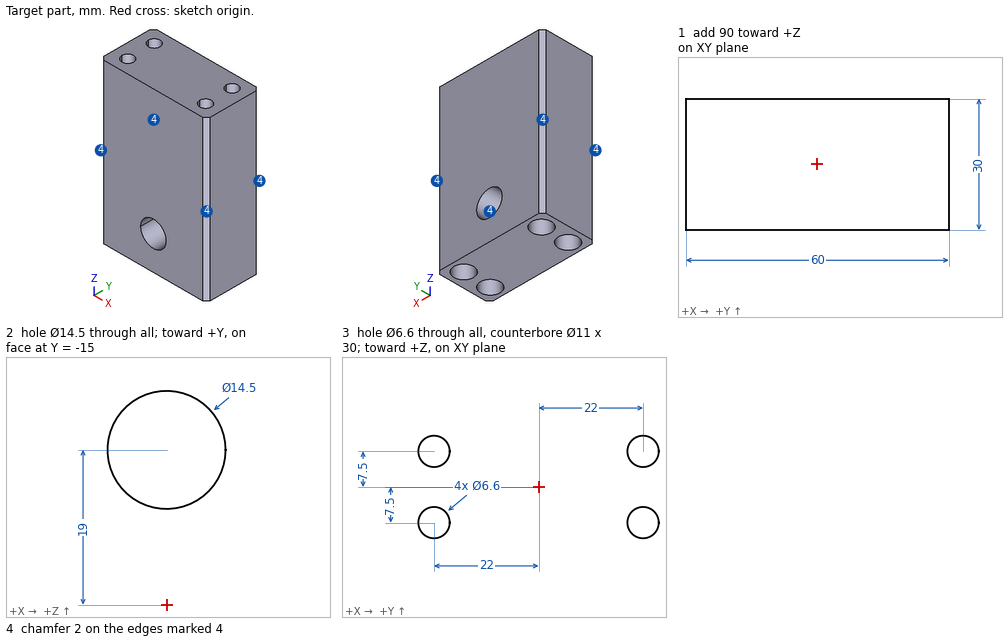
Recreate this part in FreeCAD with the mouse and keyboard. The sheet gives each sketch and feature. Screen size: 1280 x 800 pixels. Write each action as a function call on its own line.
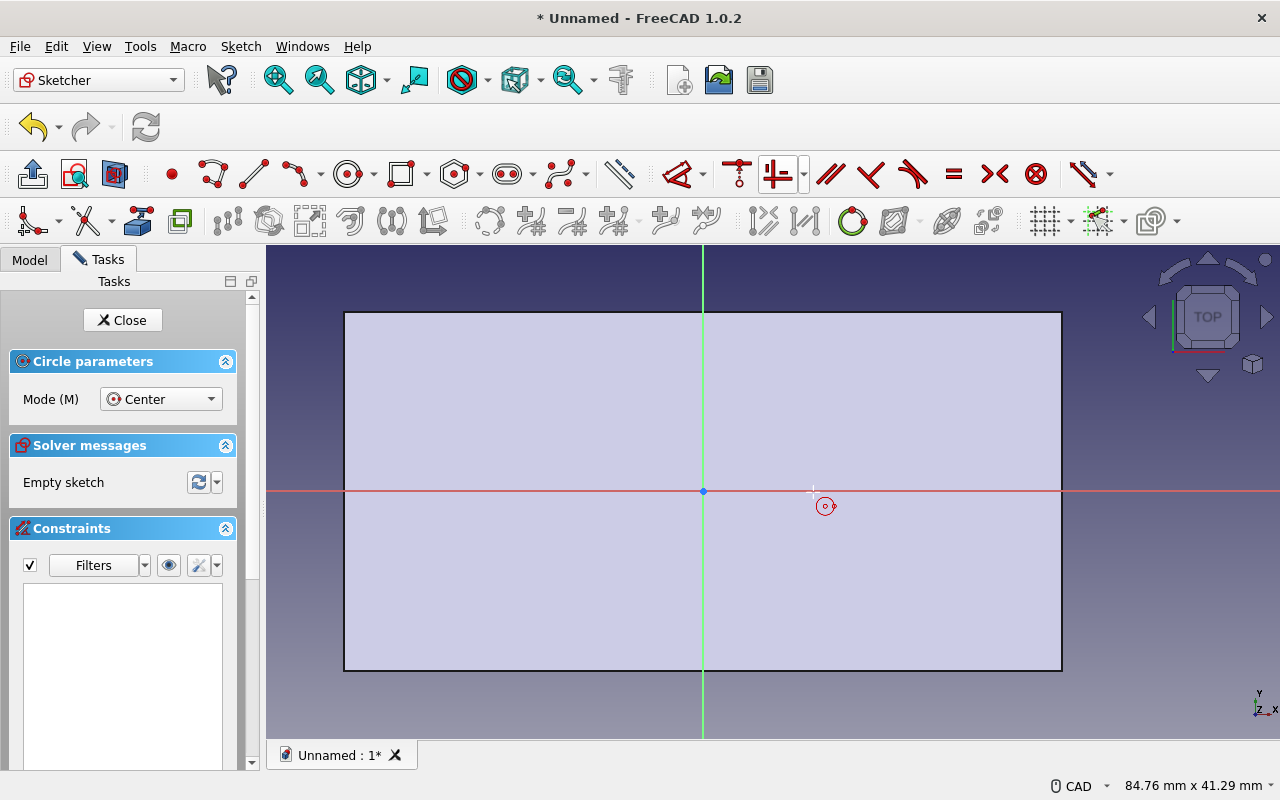
click(440, 581)
click(468, 553)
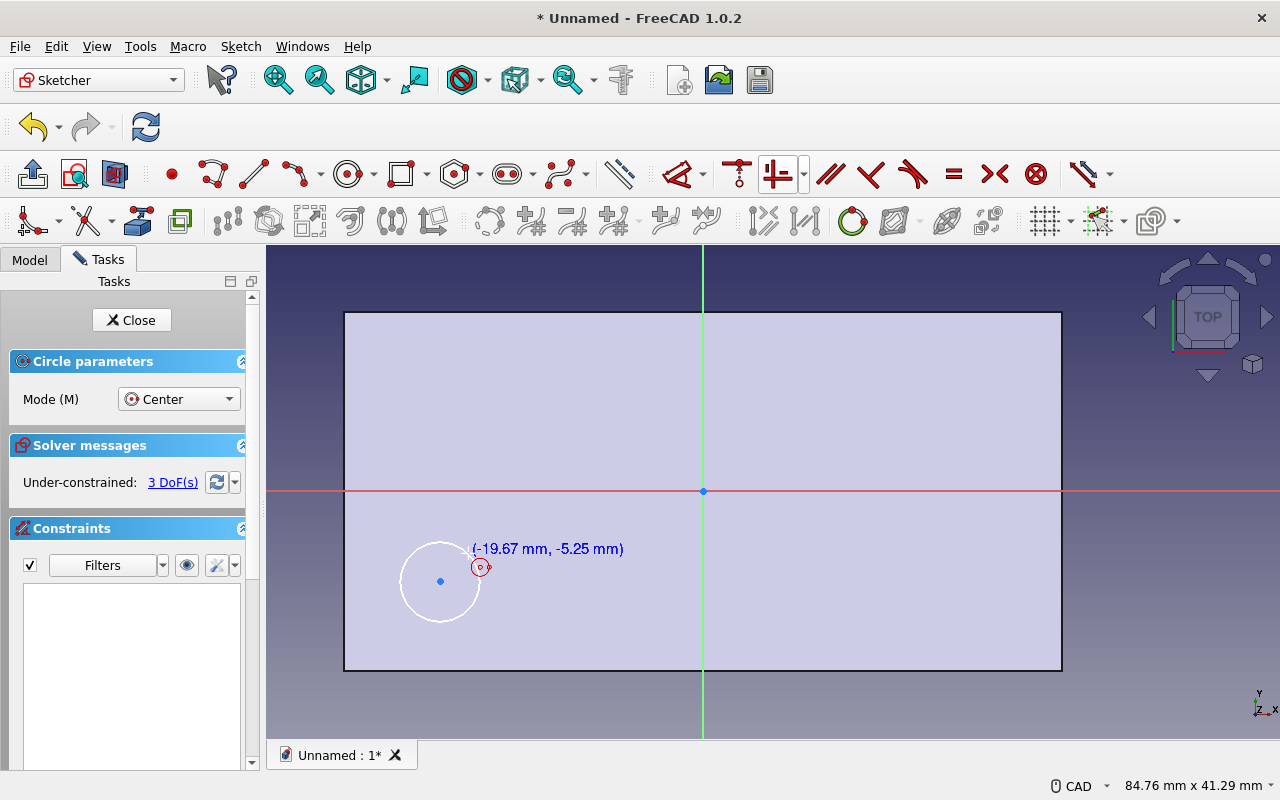
click(440, 401)
click(468, 374)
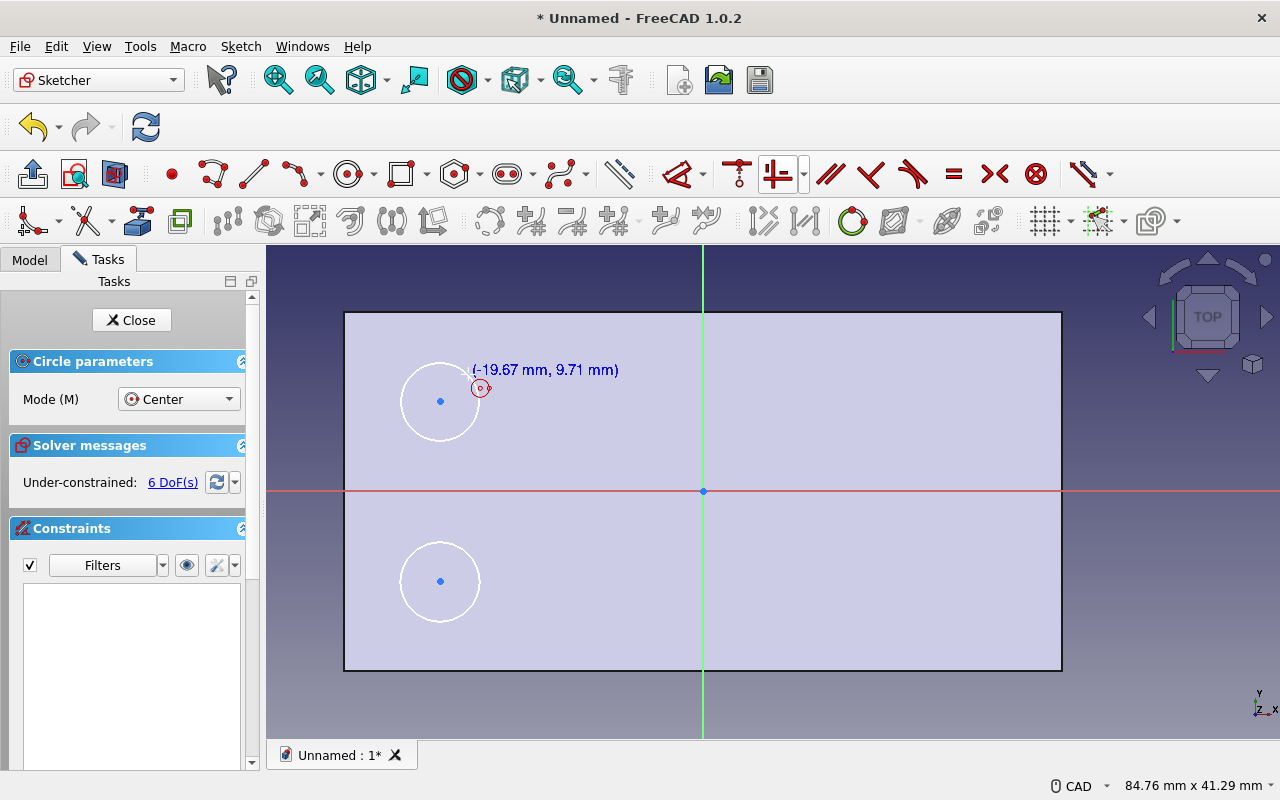
click(967, 401)
click(994, 374)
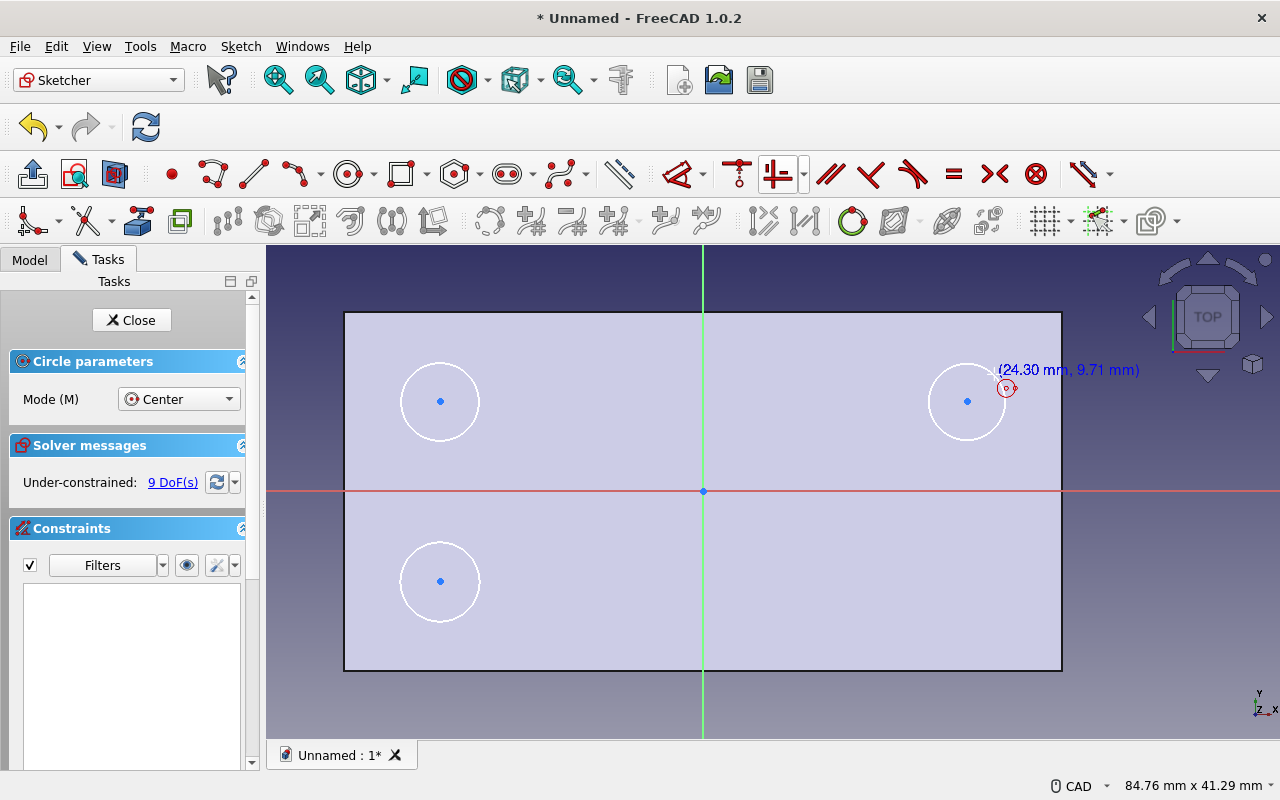
click(967, 581)
click(994, 553)
key(Escape)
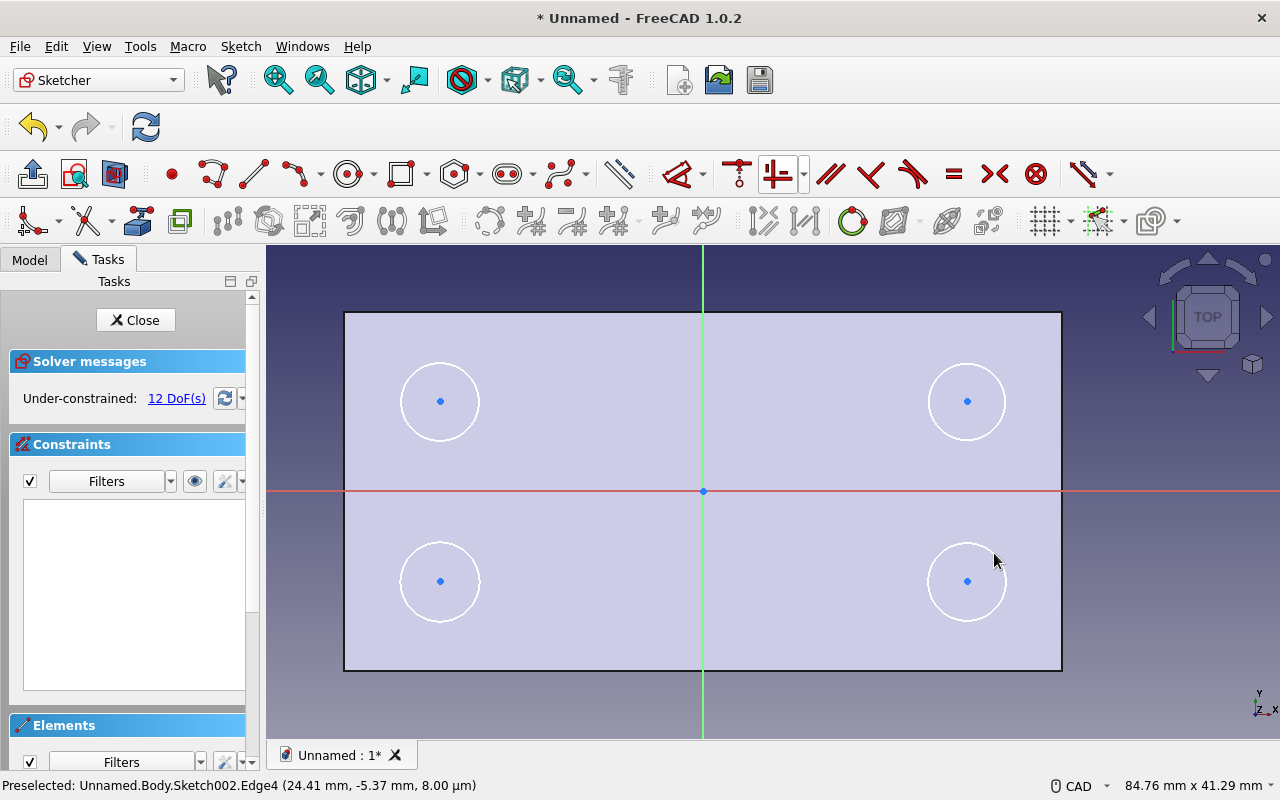
click(468, 554)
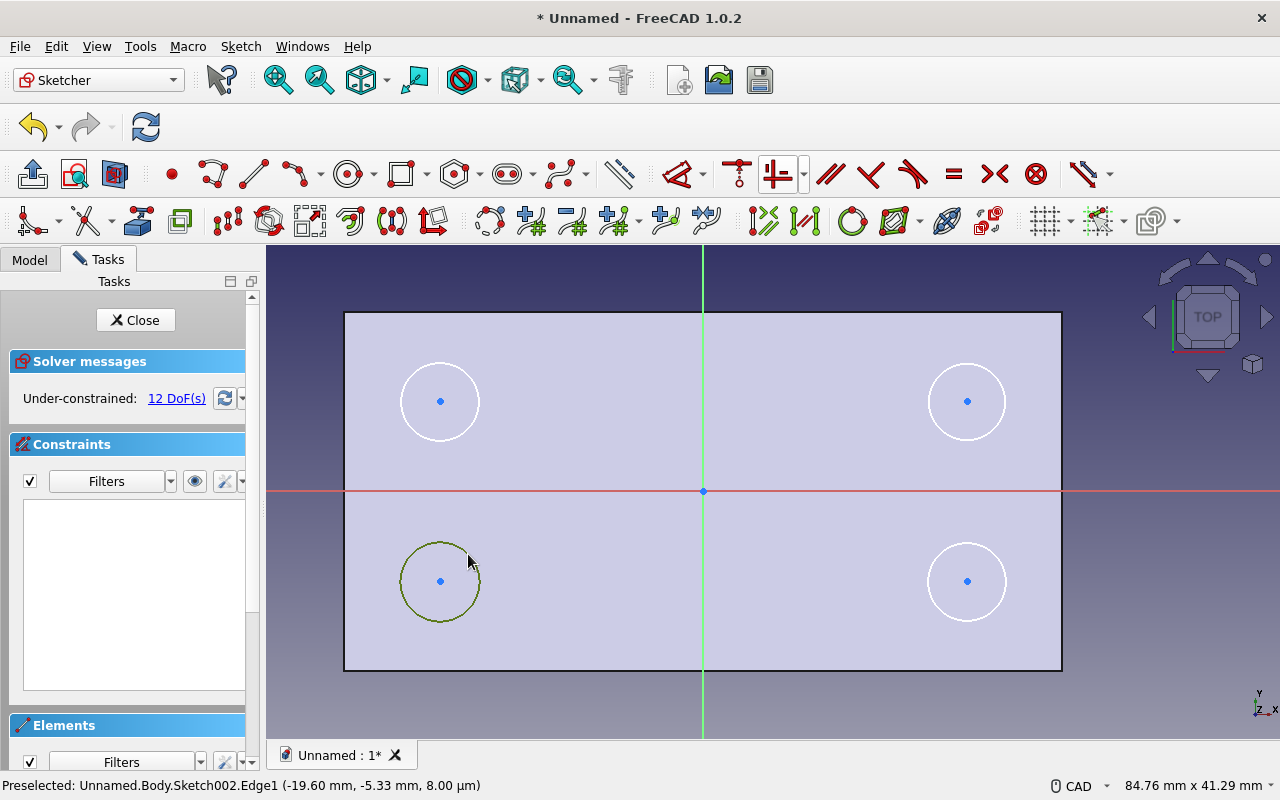
click(467, 374)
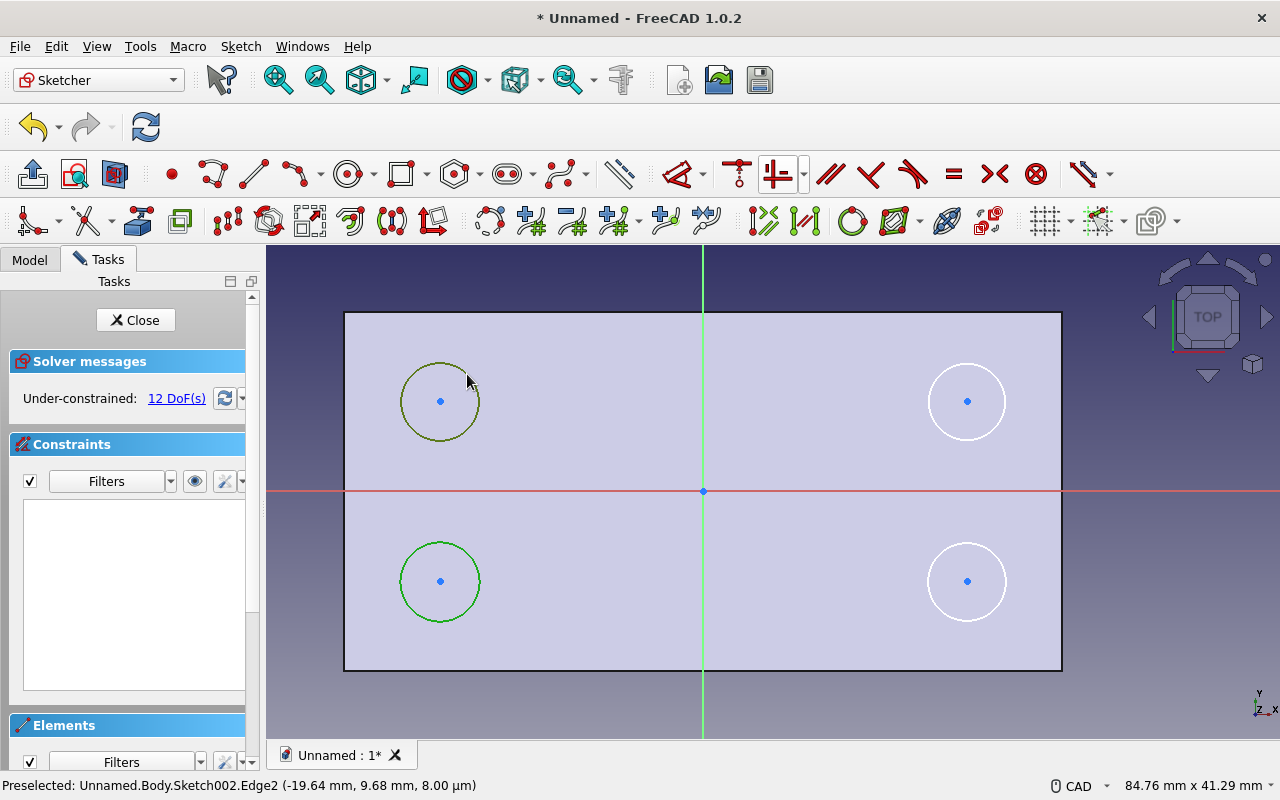
click(994, 375)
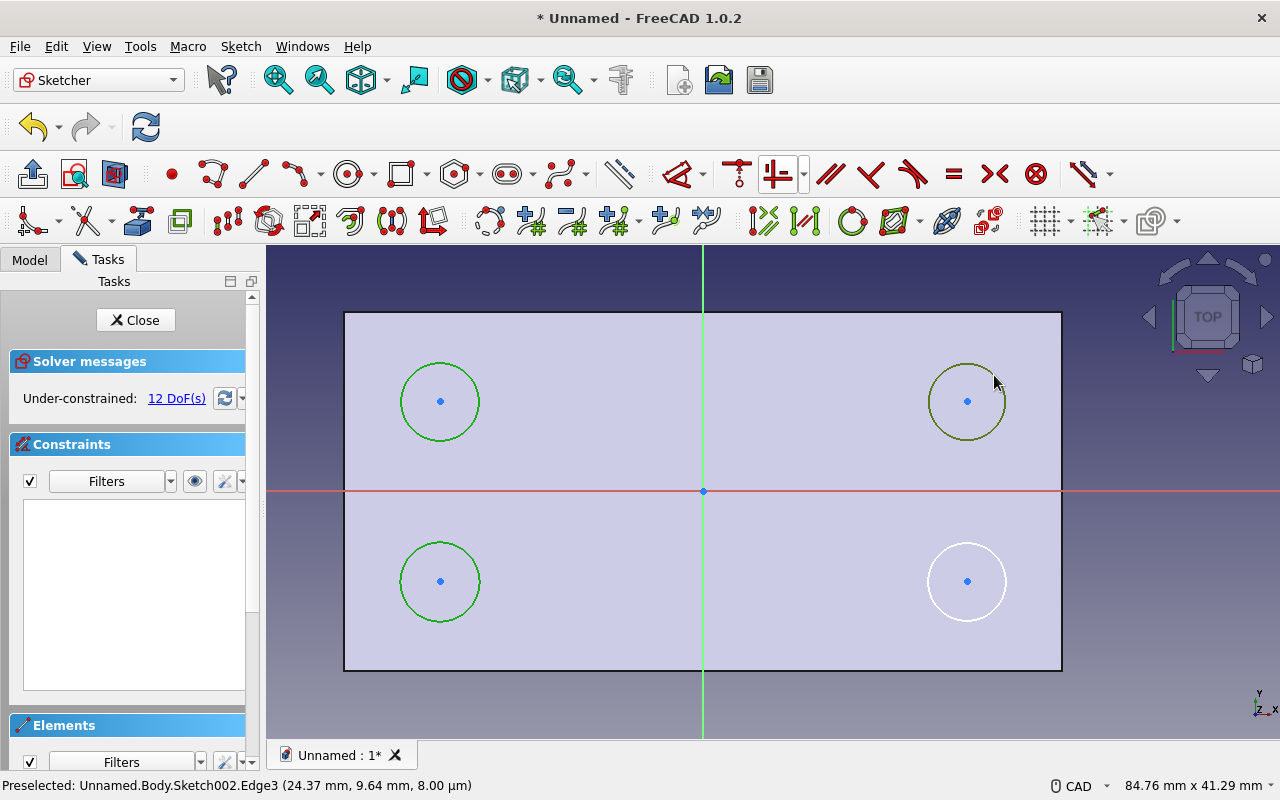
click(994, 554)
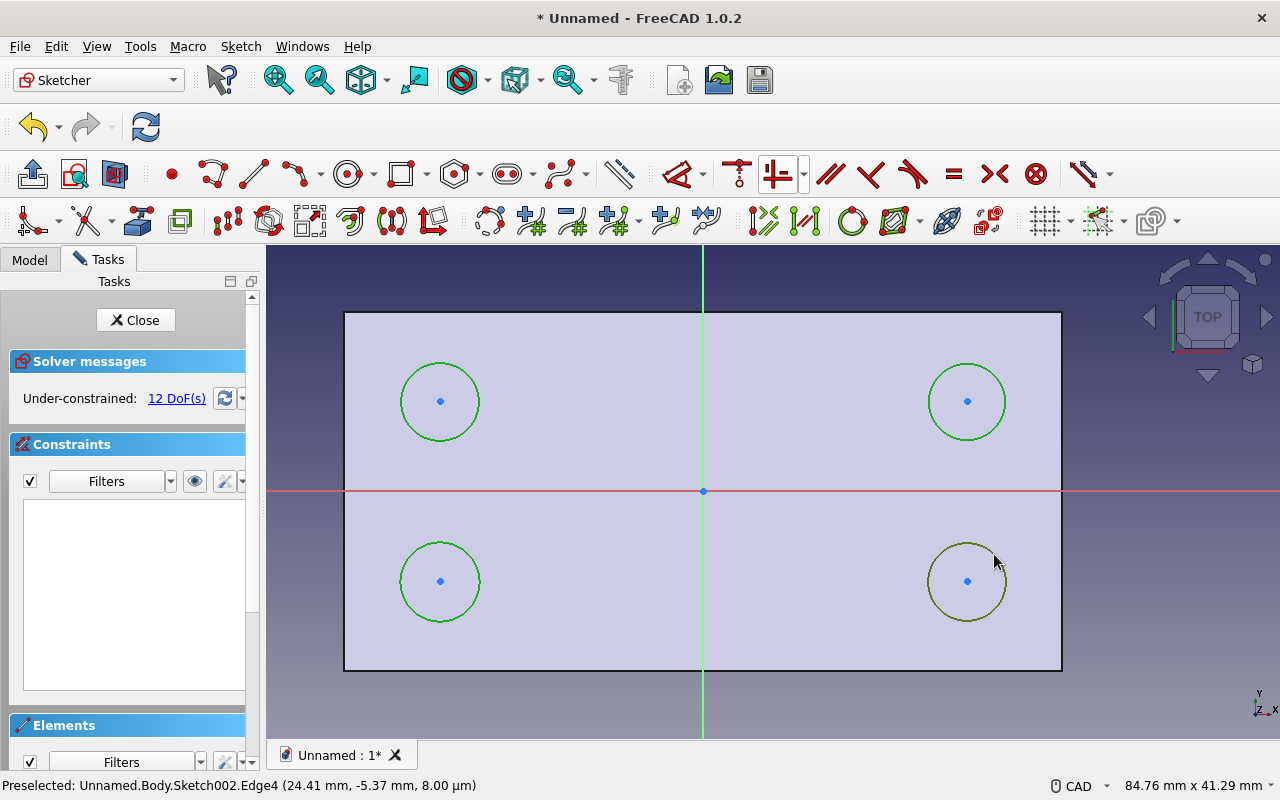
key(e)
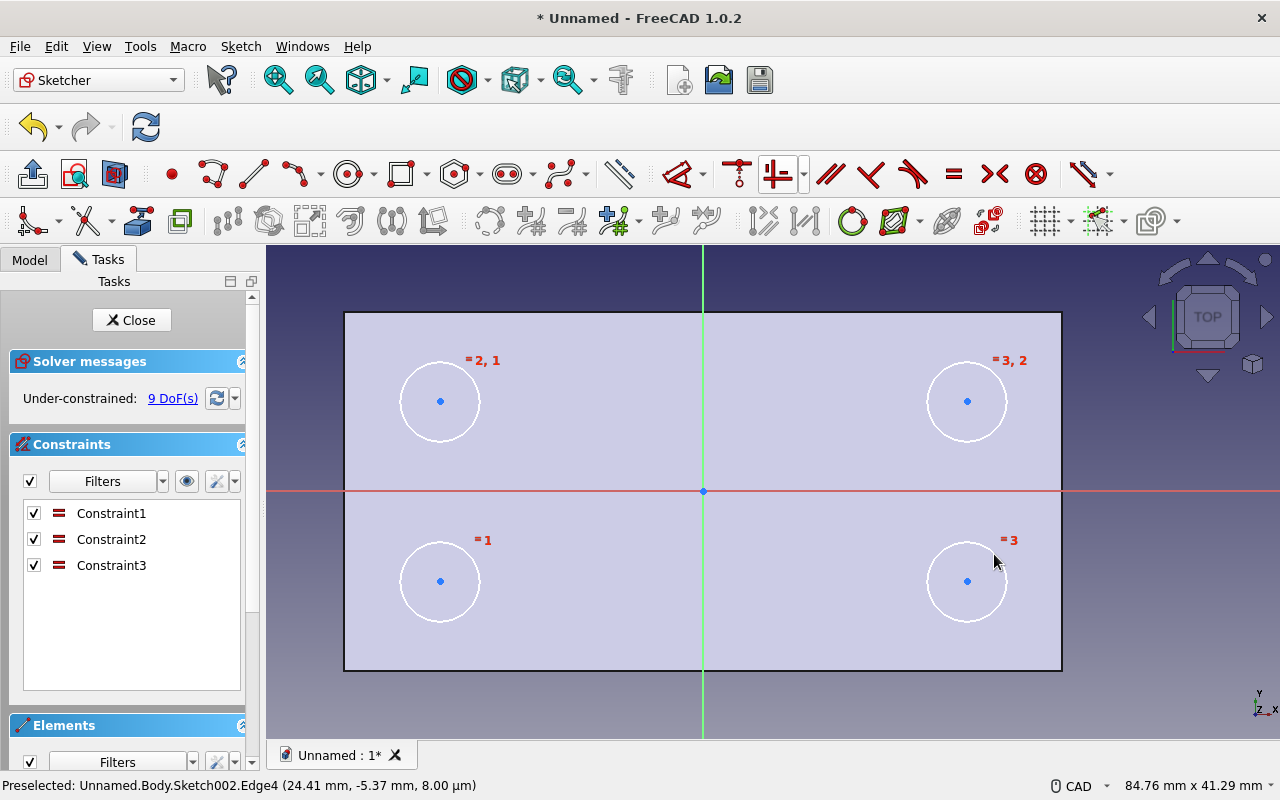
click(440, 582)